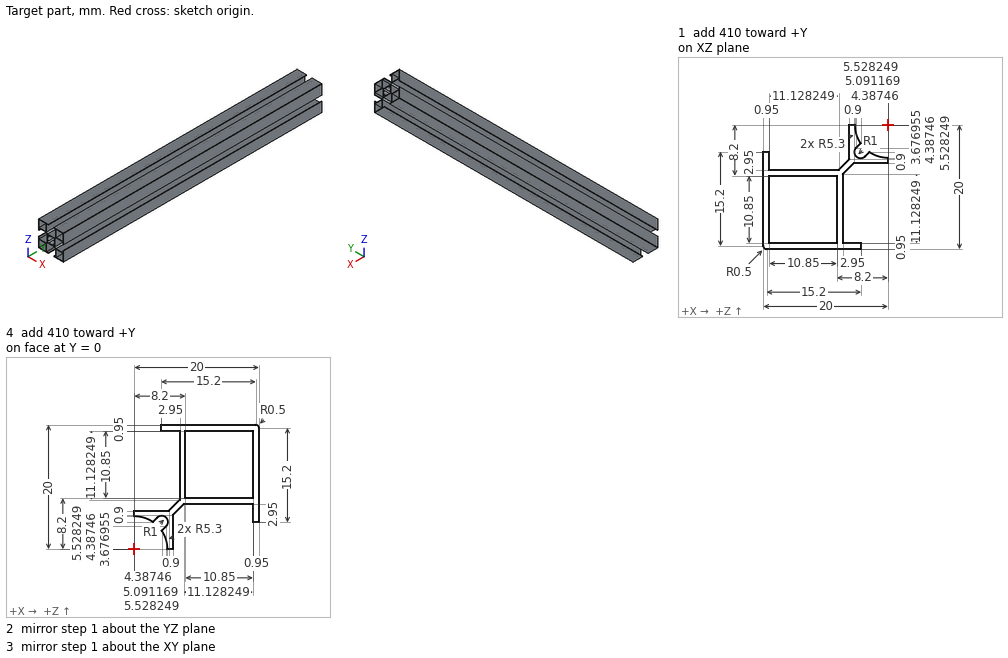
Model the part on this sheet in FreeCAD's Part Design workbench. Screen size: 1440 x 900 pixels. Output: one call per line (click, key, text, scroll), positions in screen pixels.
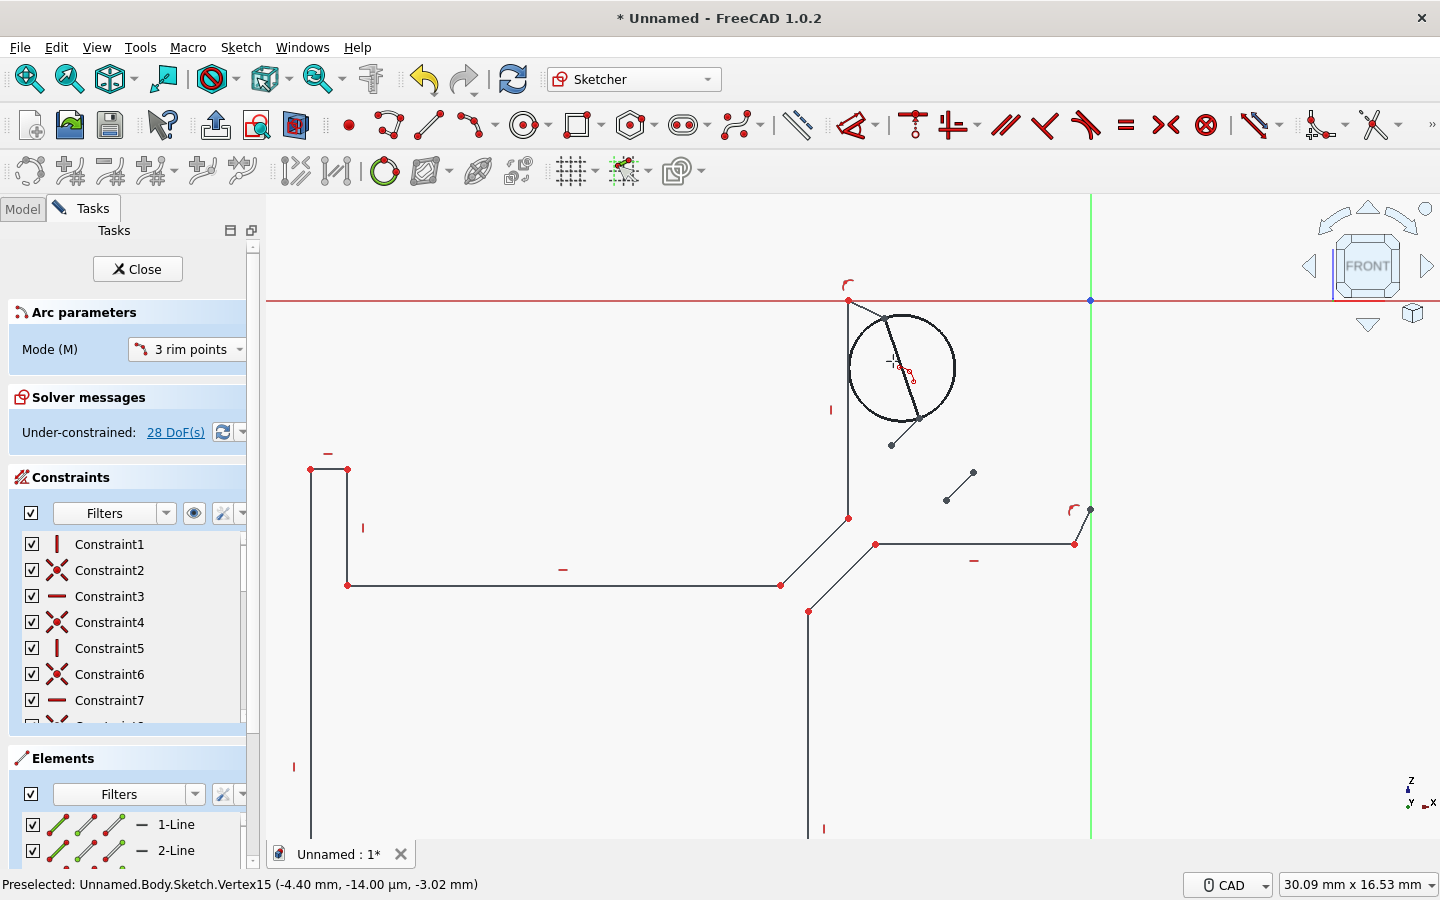
click(893, 361)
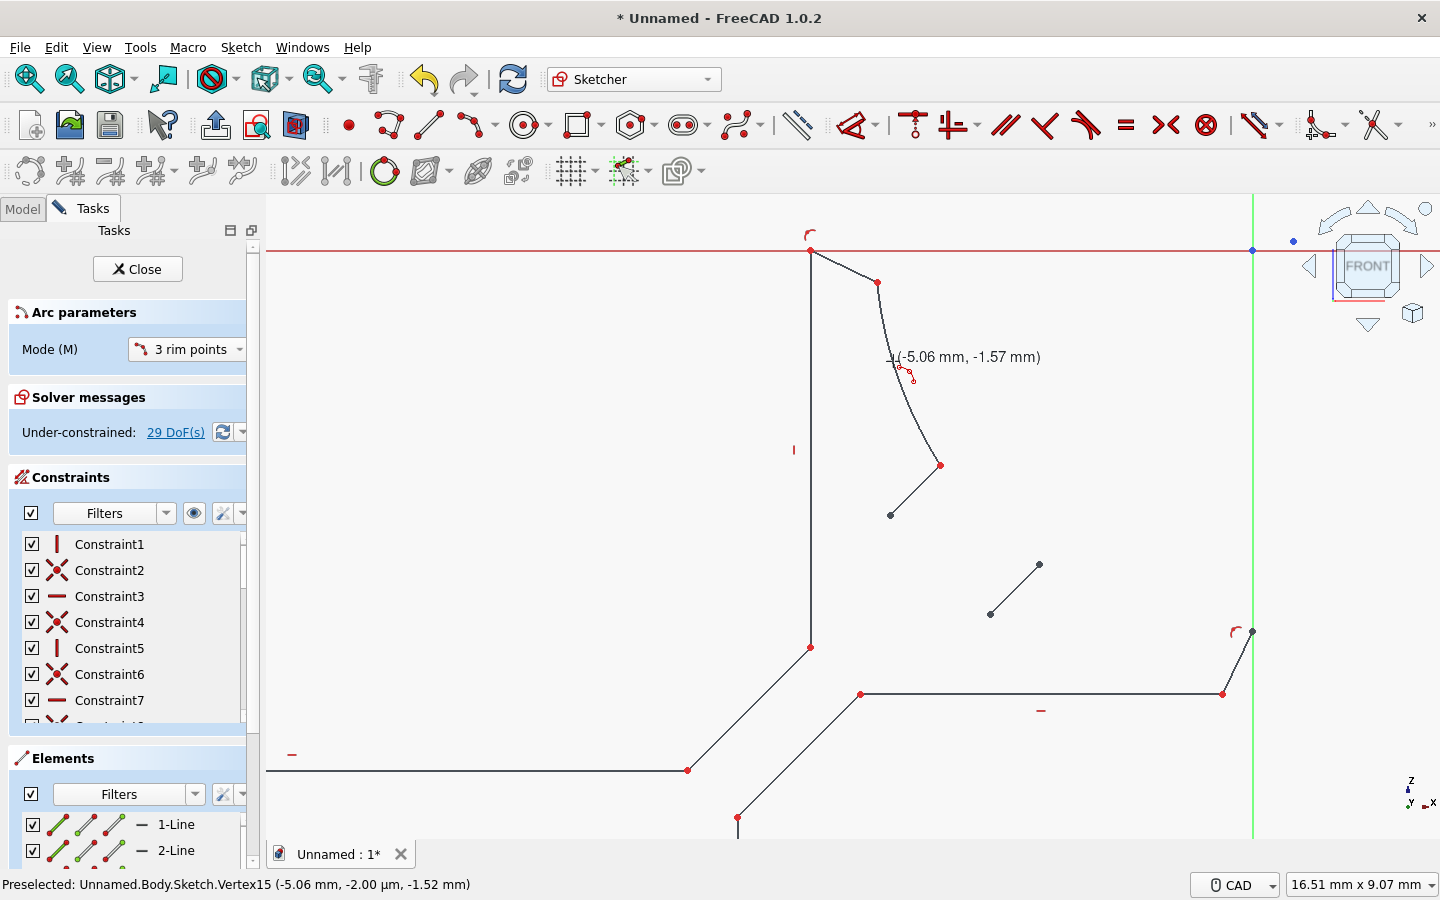
click(890, 515)
click(990, 615)
click(891, 613)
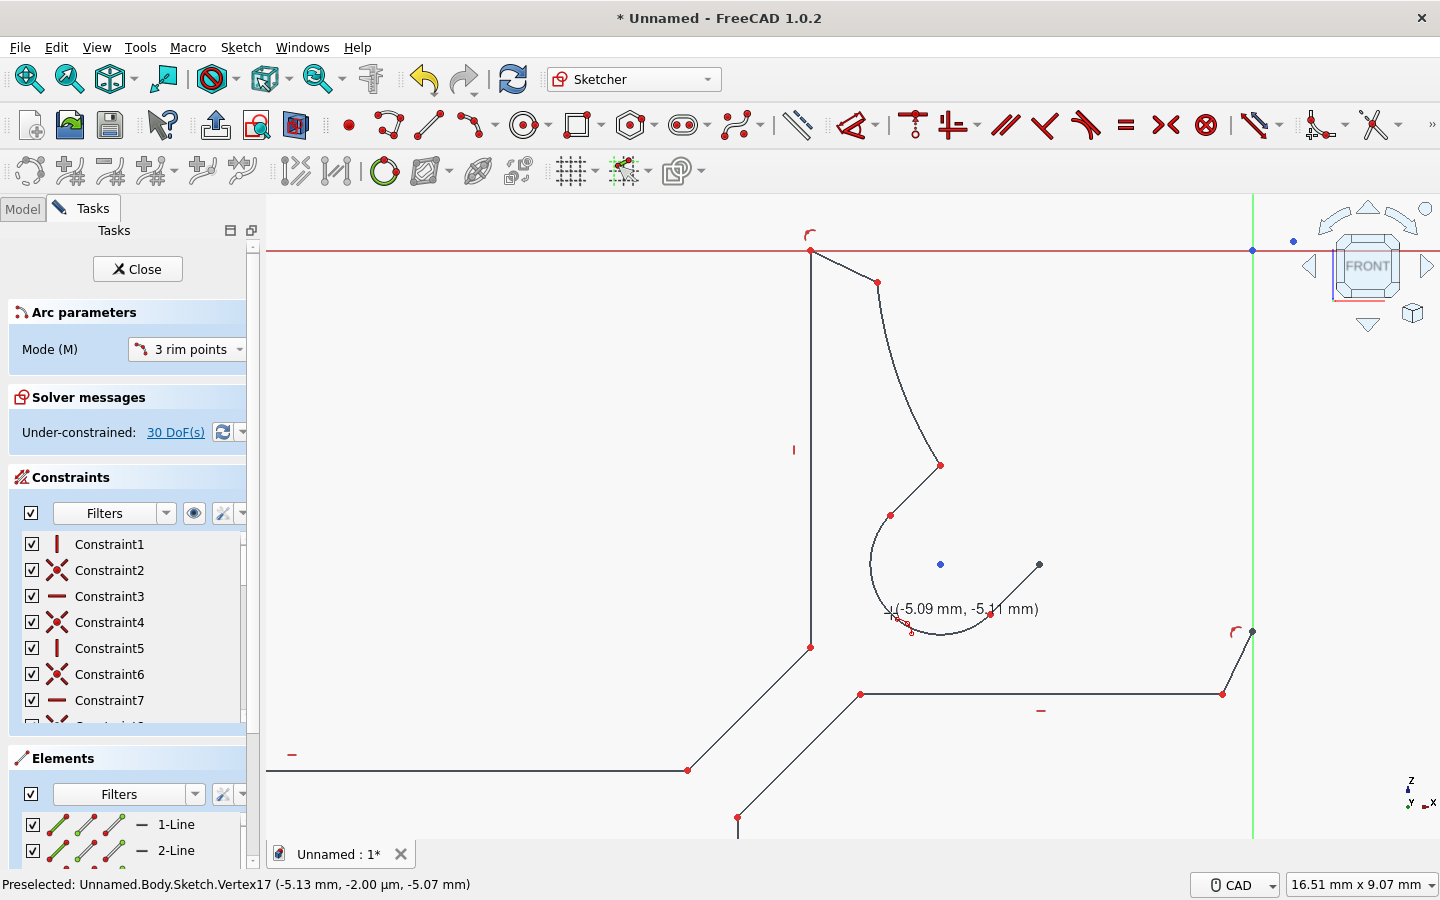
click(1040, 565)
click(1253, 631)
click(1142, 611)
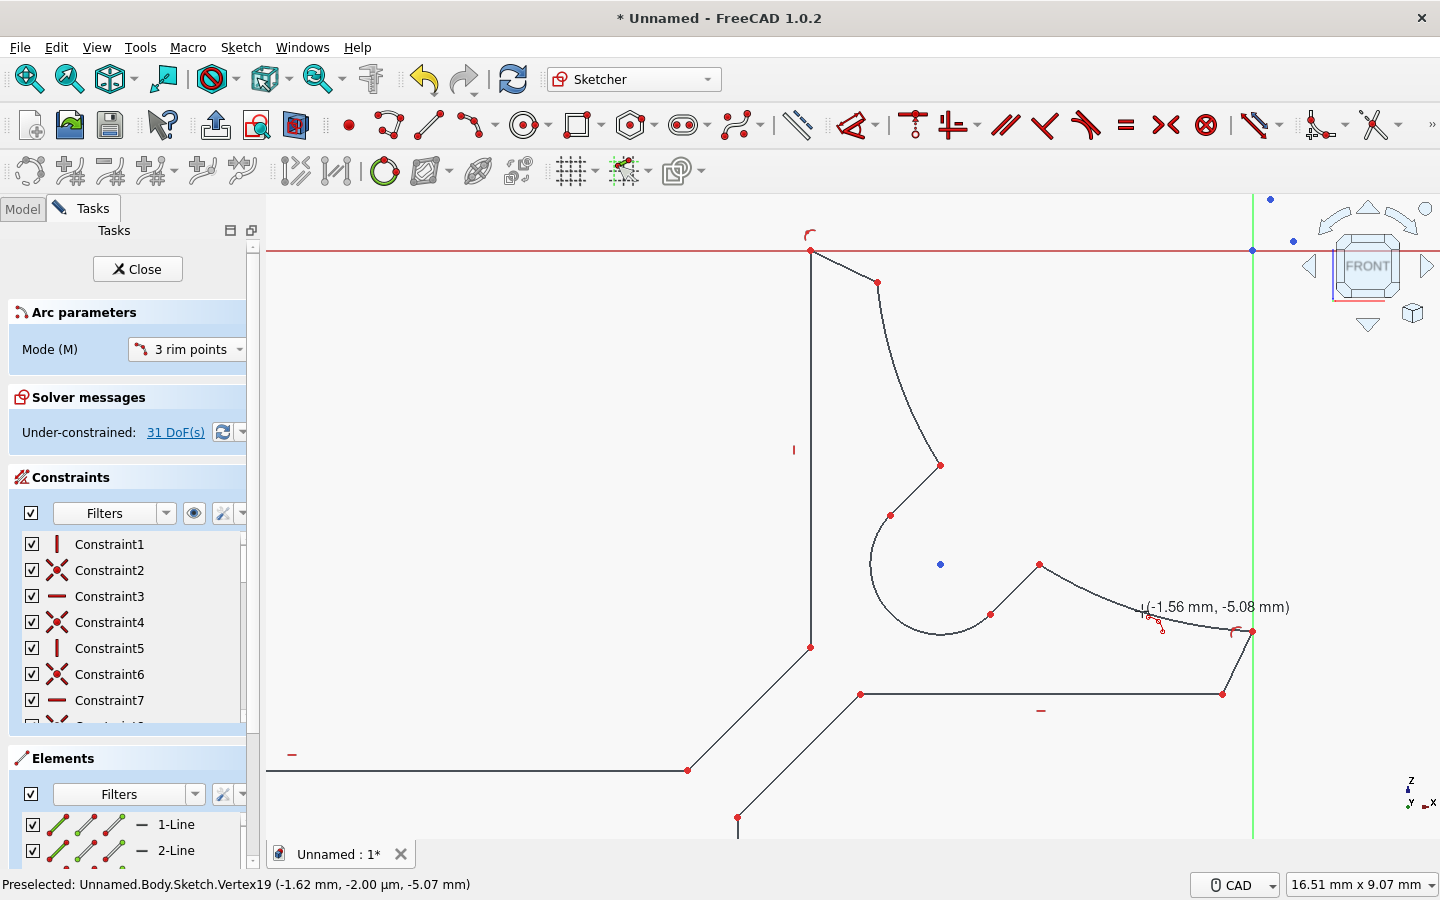
scroll(889, 325, down, 6)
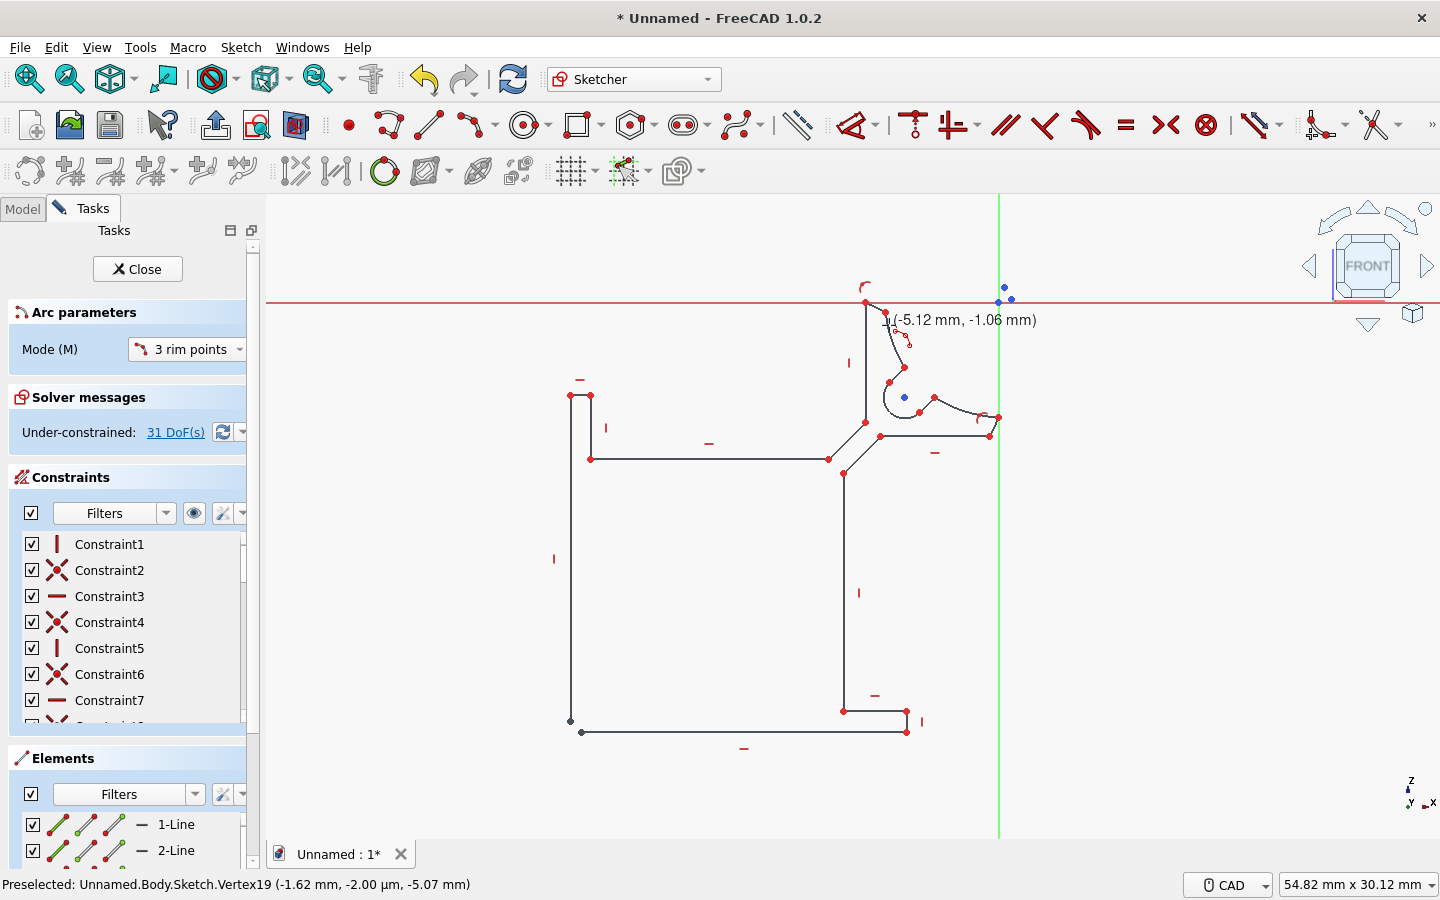
click(582, 732)
click(571, 721)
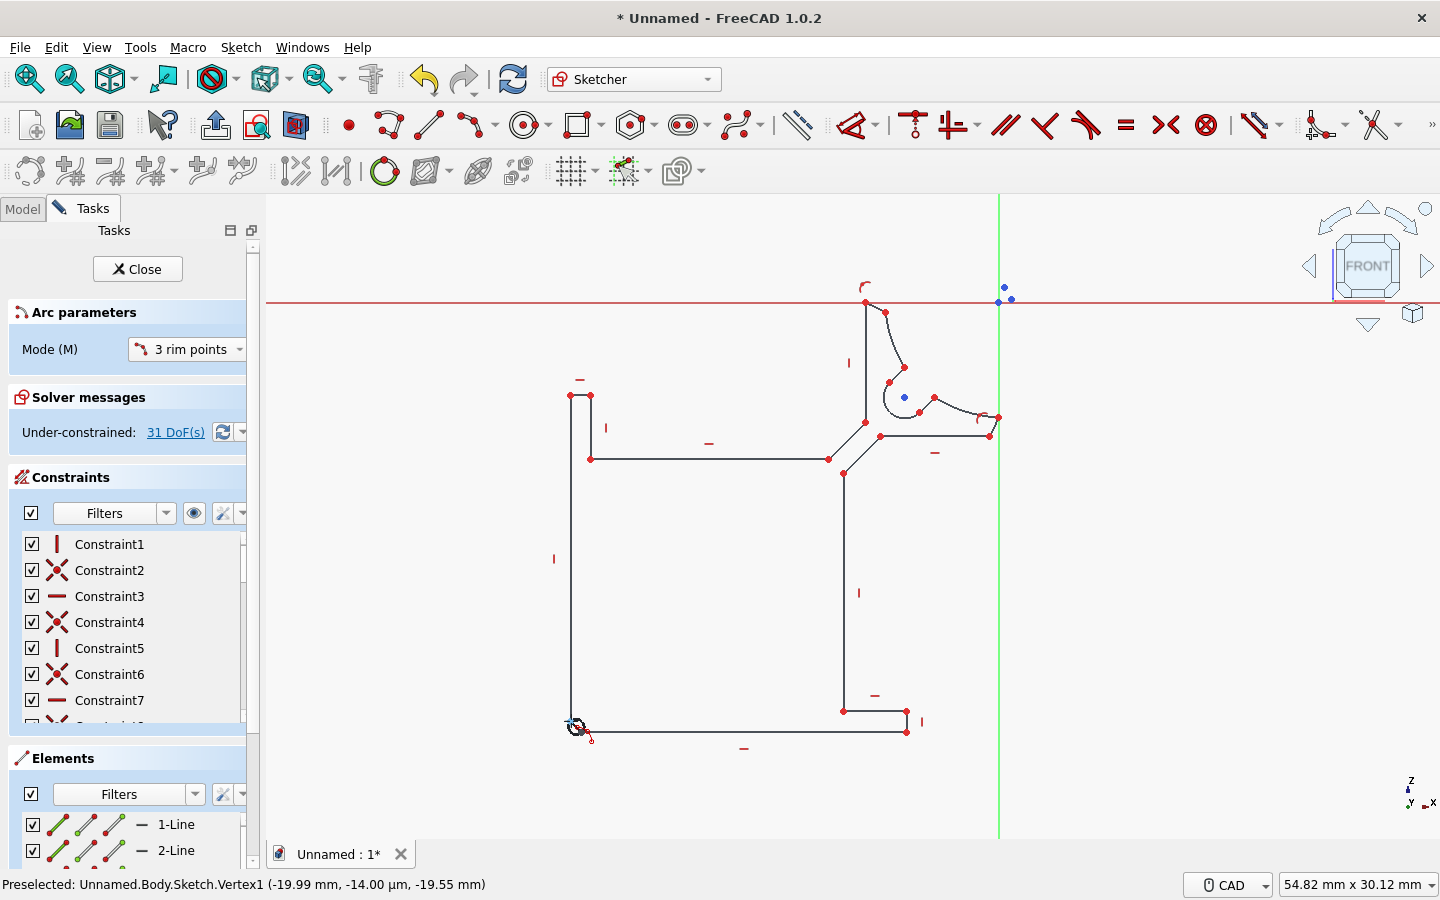
scroll(574, 728, up, 9)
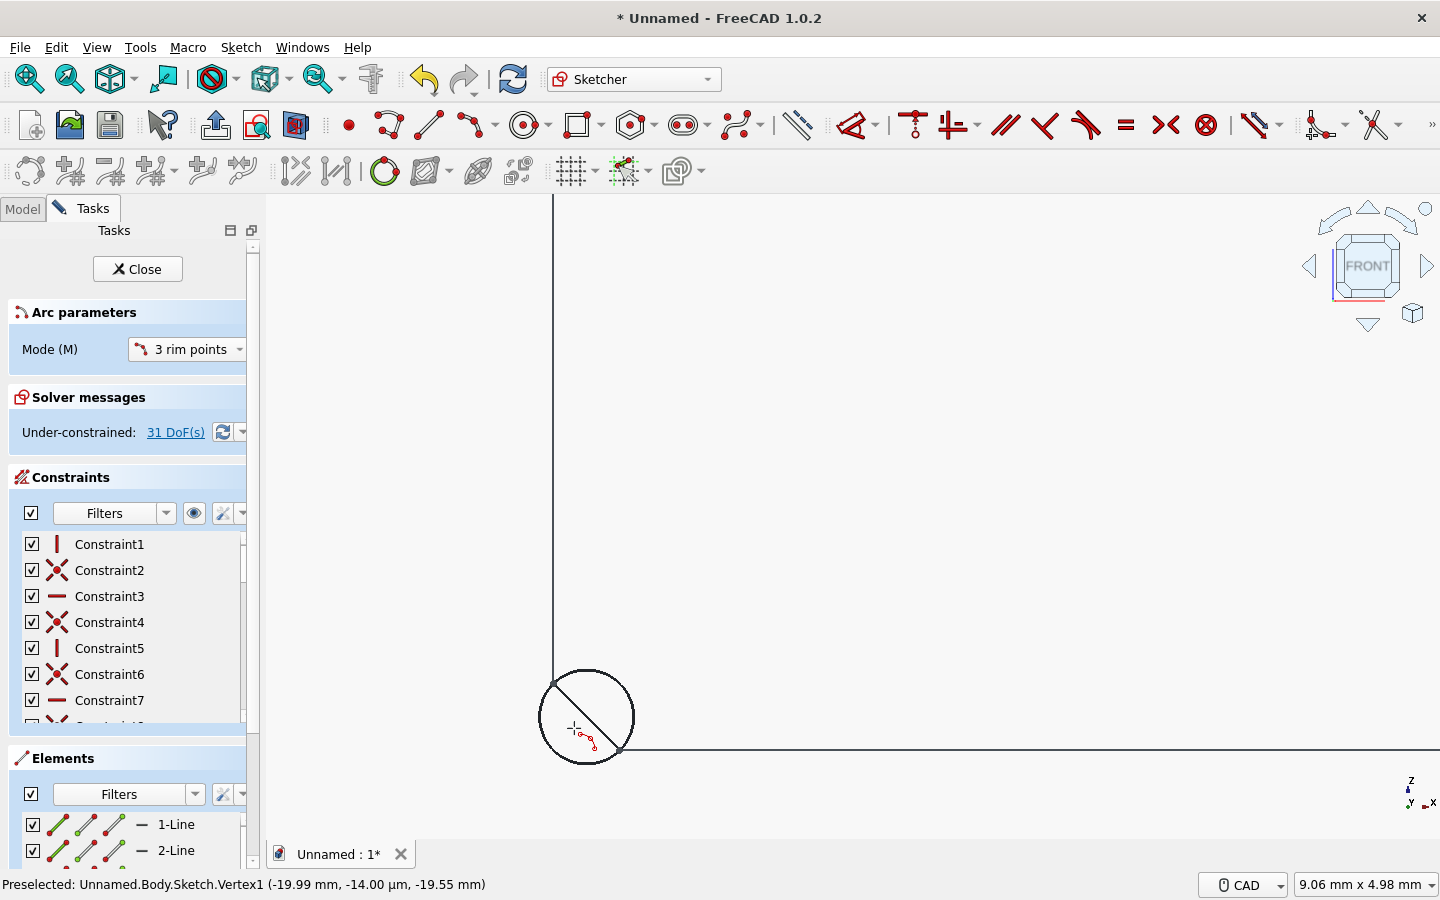
click(571, 723)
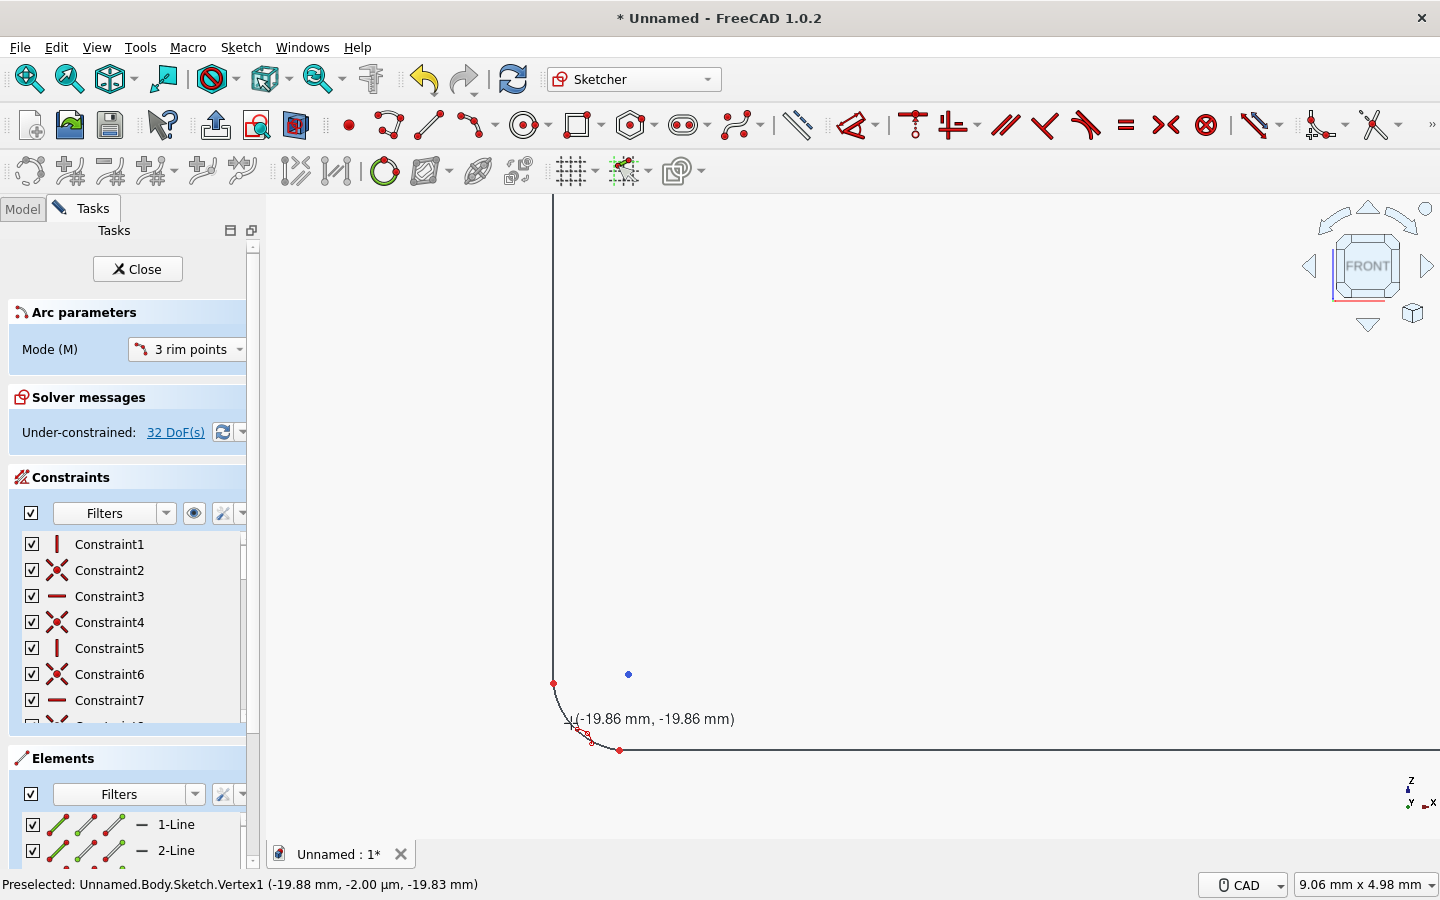
click(578, 126)